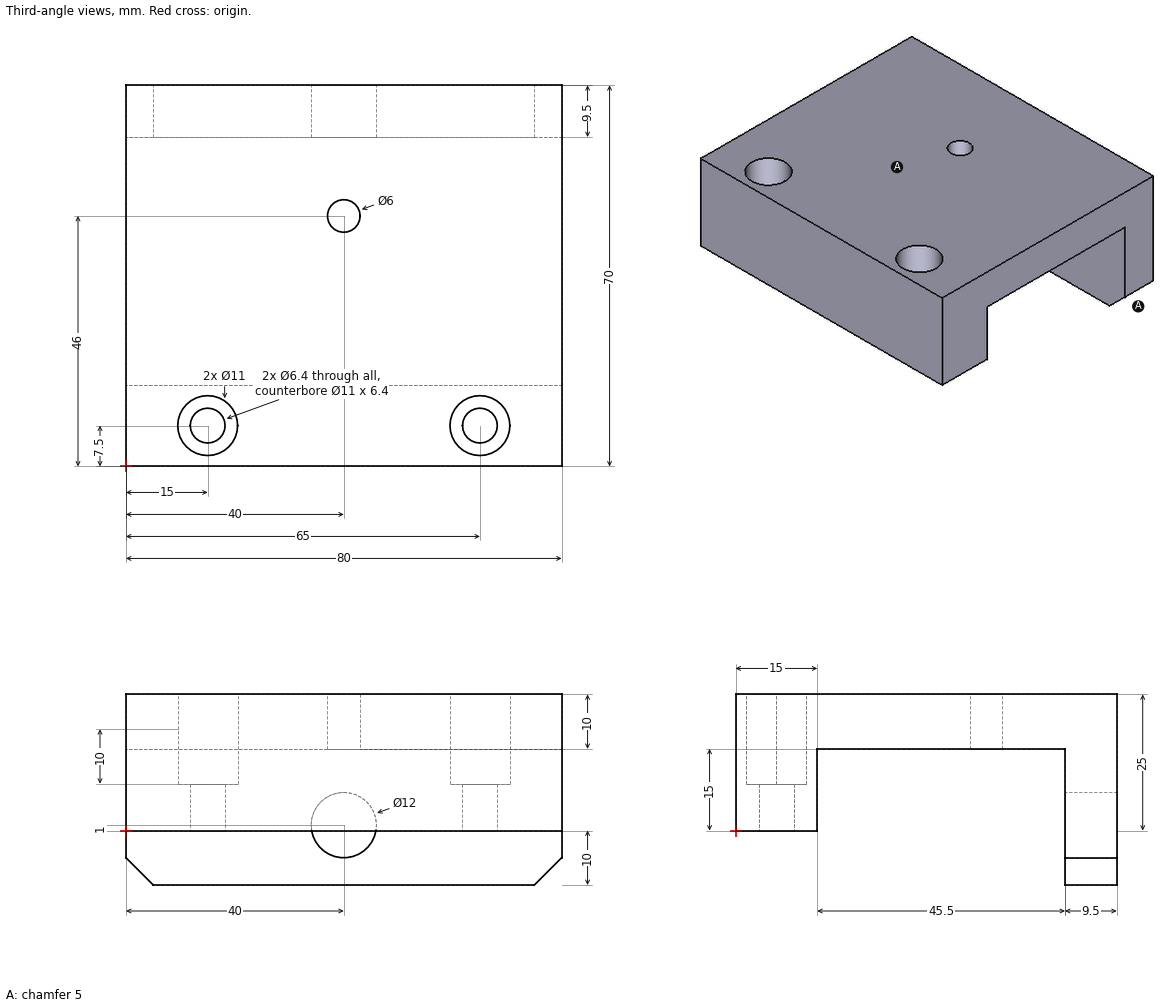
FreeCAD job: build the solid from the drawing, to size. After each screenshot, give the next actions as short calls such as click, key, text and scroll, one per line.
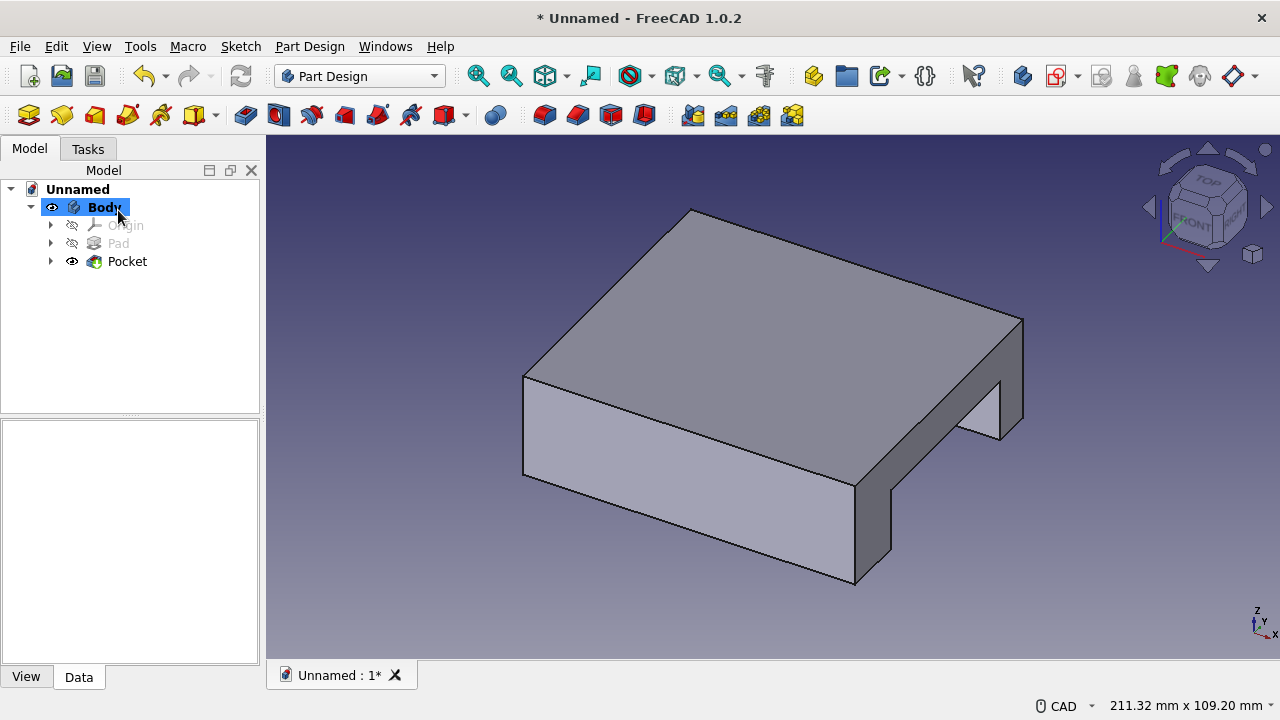
click(773, 347)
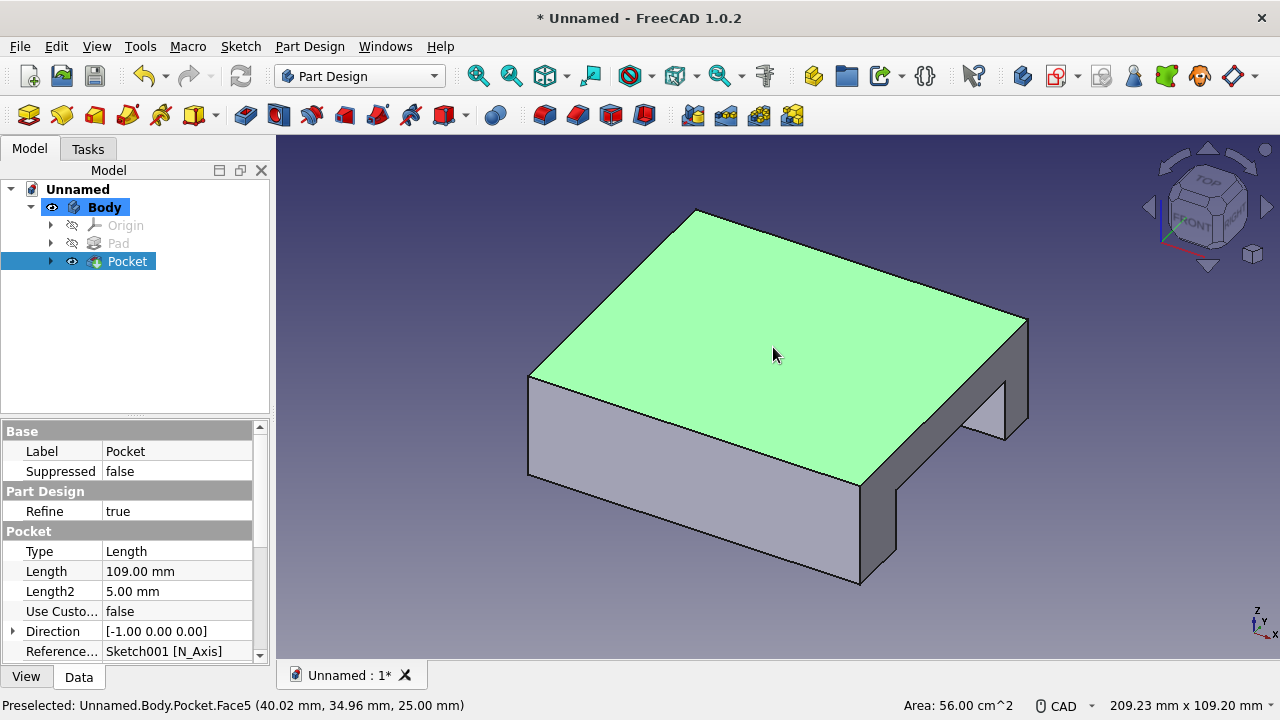
click(1056, 76)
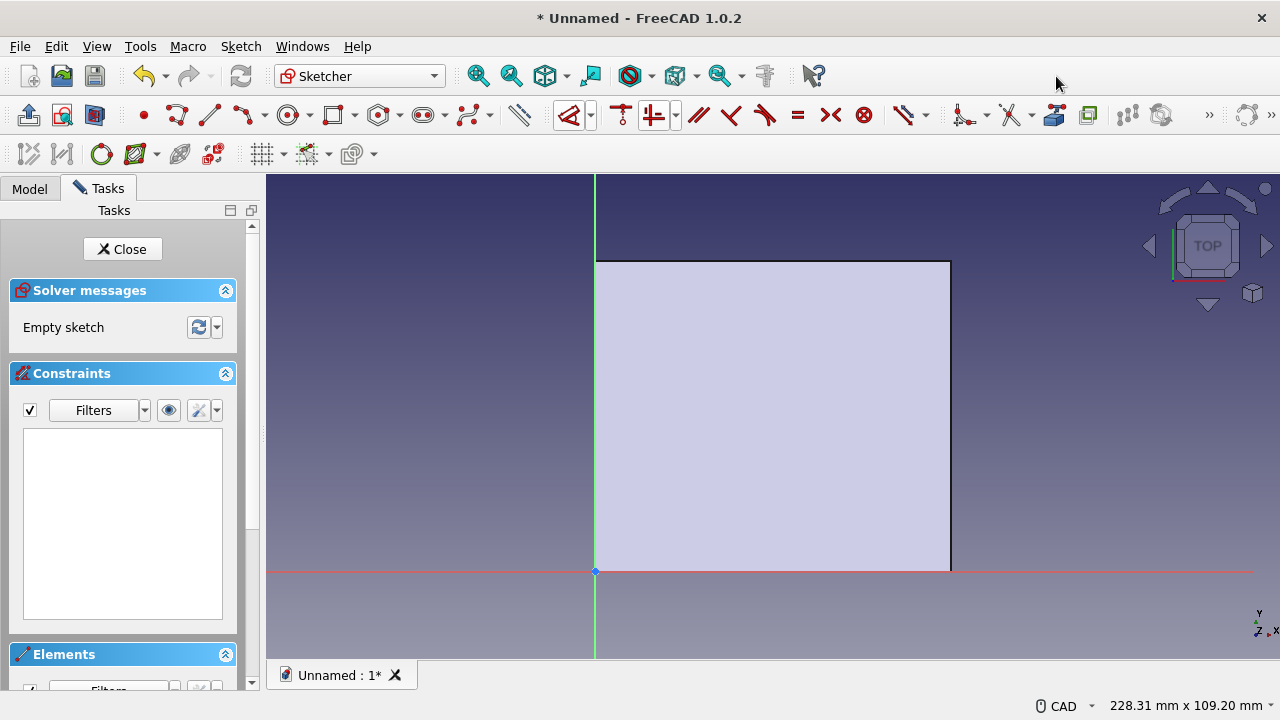
scroll(798, 631, up, 3)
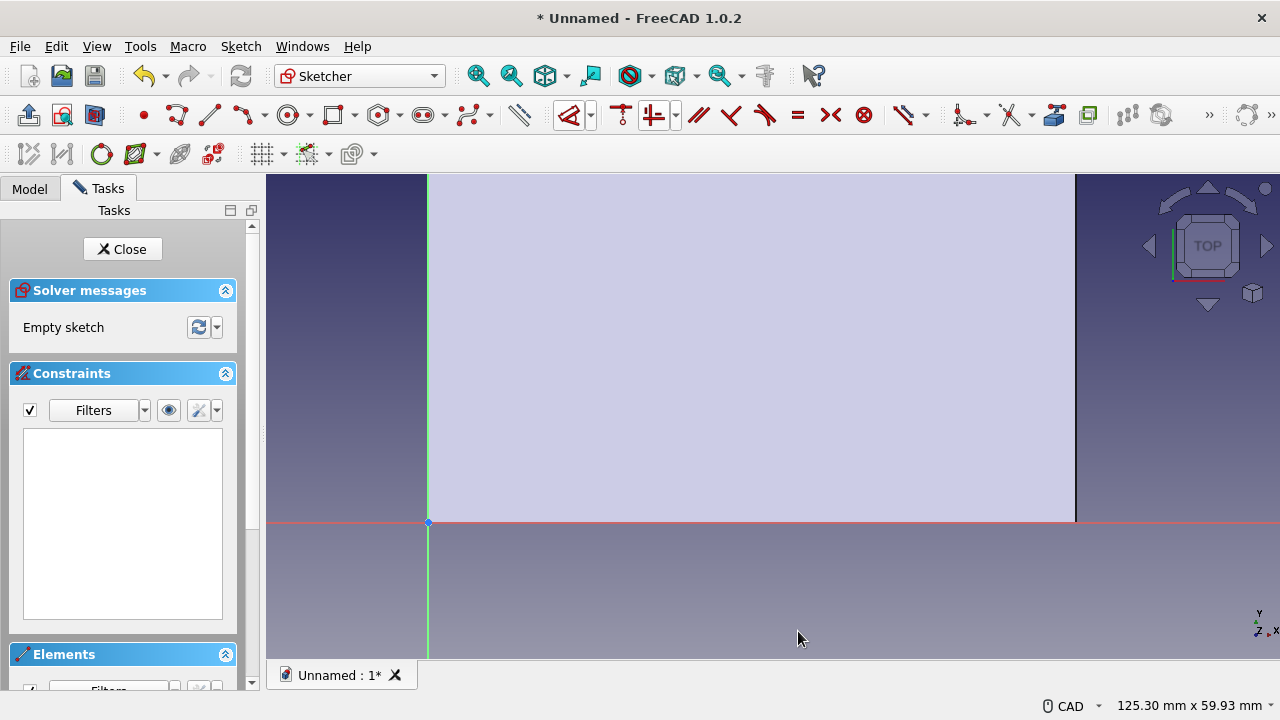
click(288, 116)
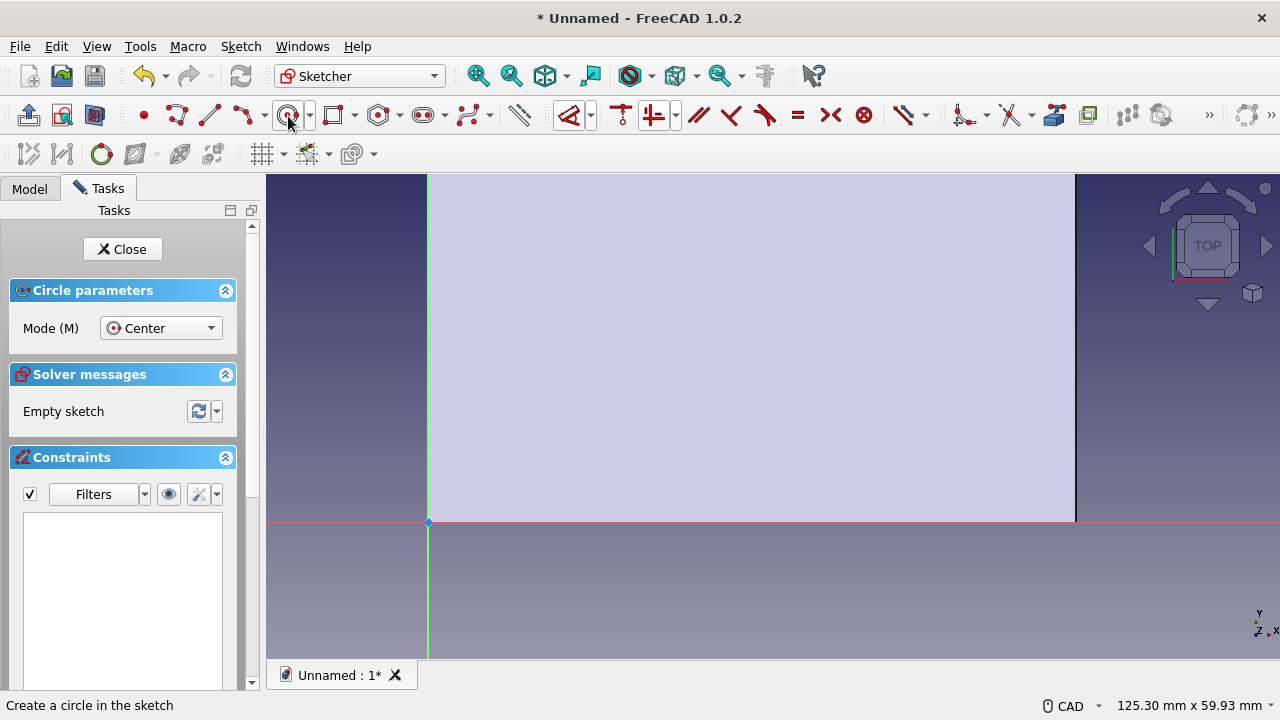
click(550, 462)
move(568, 444)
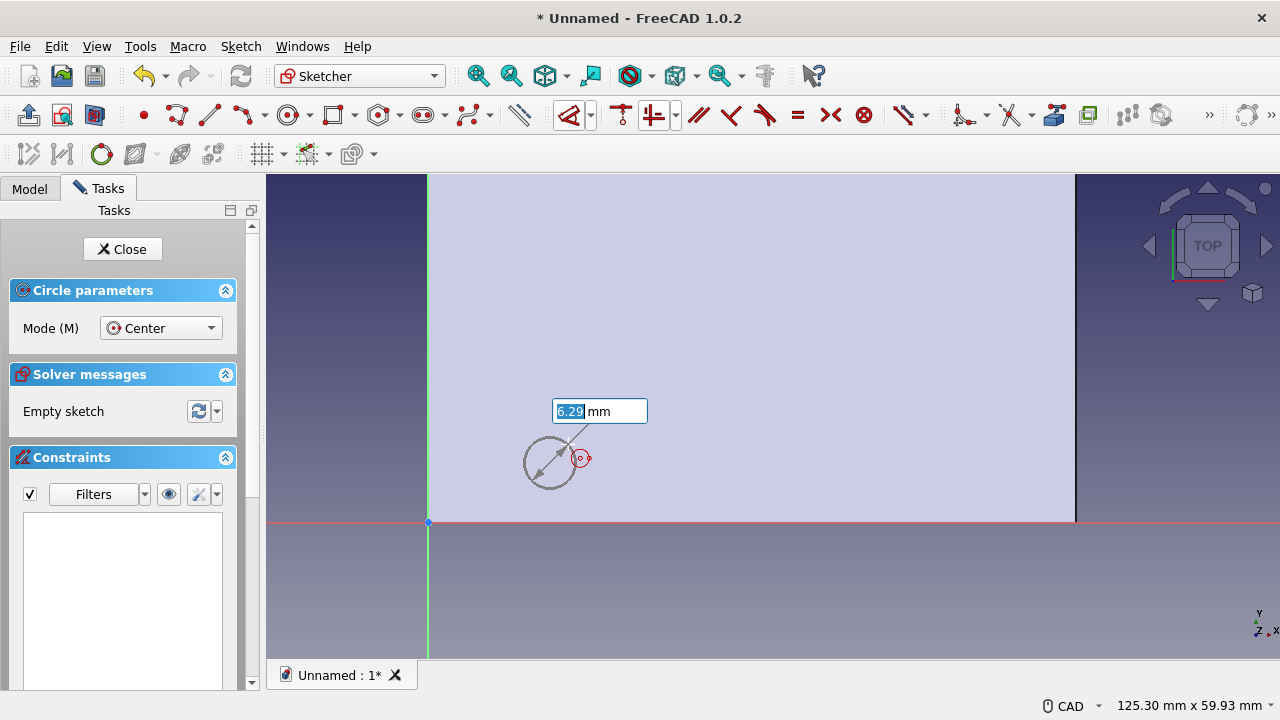
text(6.4)
key(Return)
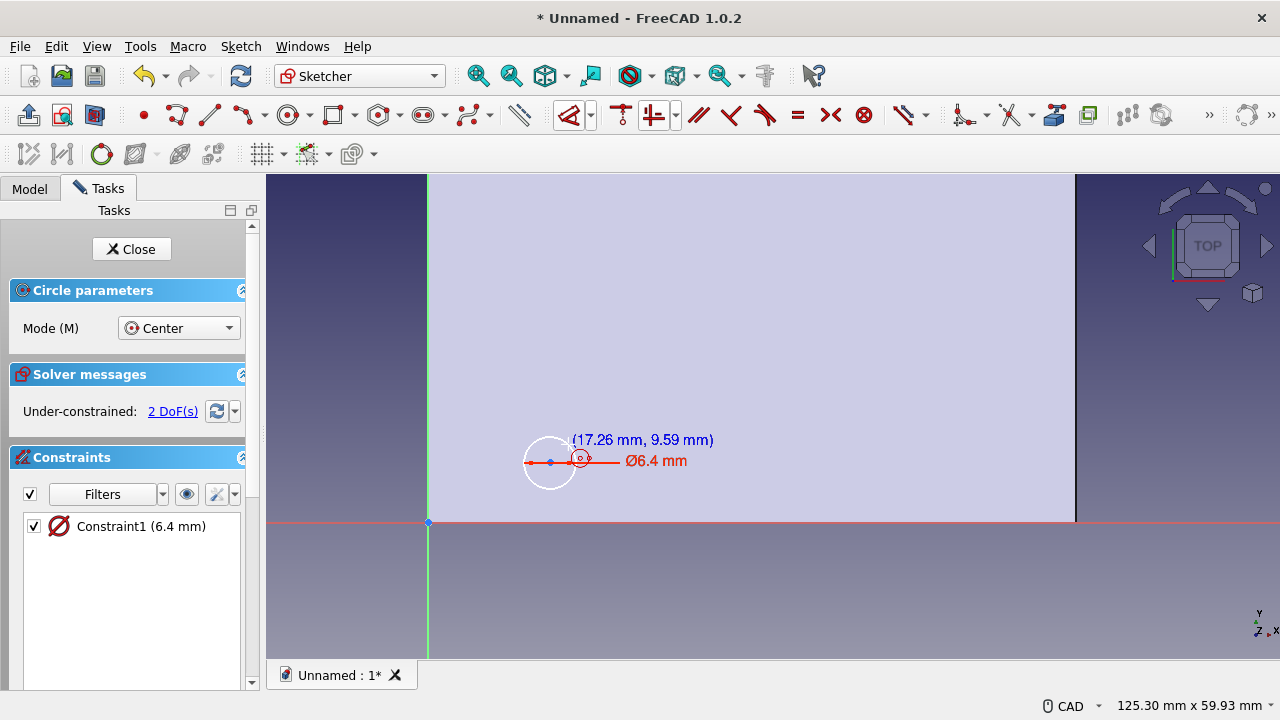
click(954, 462)
move(973, 444)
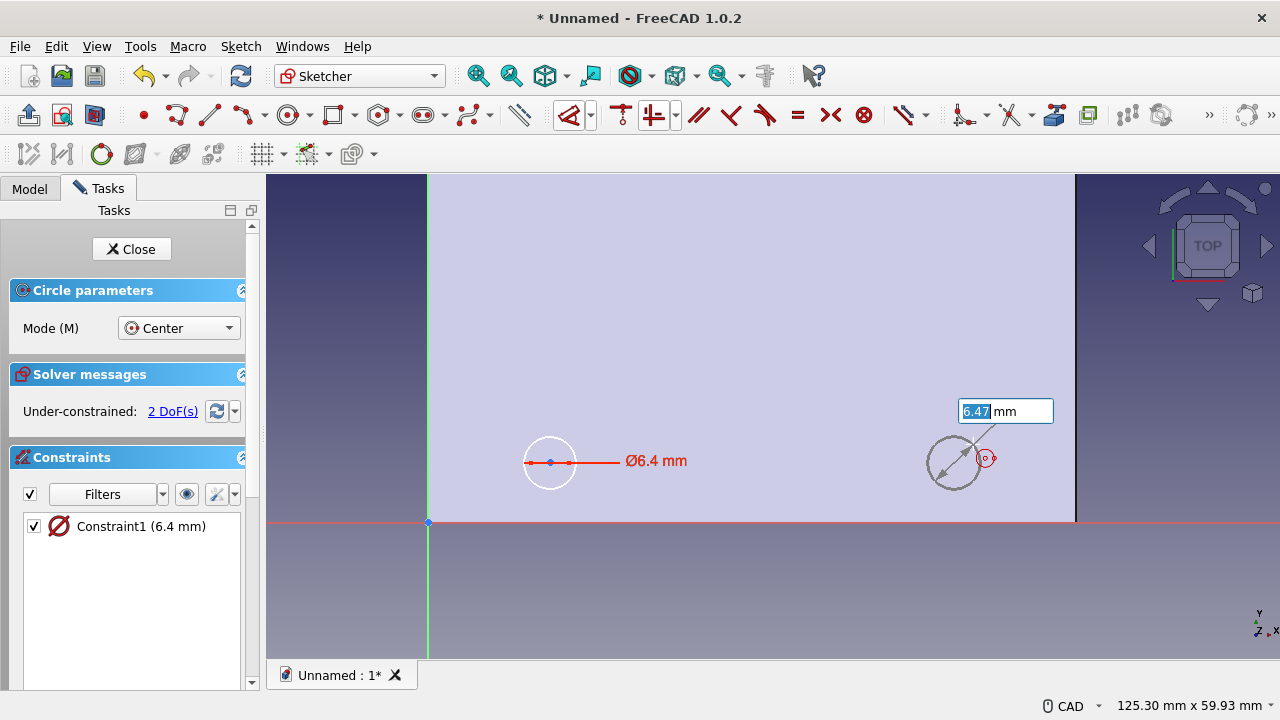
text(6.4)
key(Return)
key(Escape)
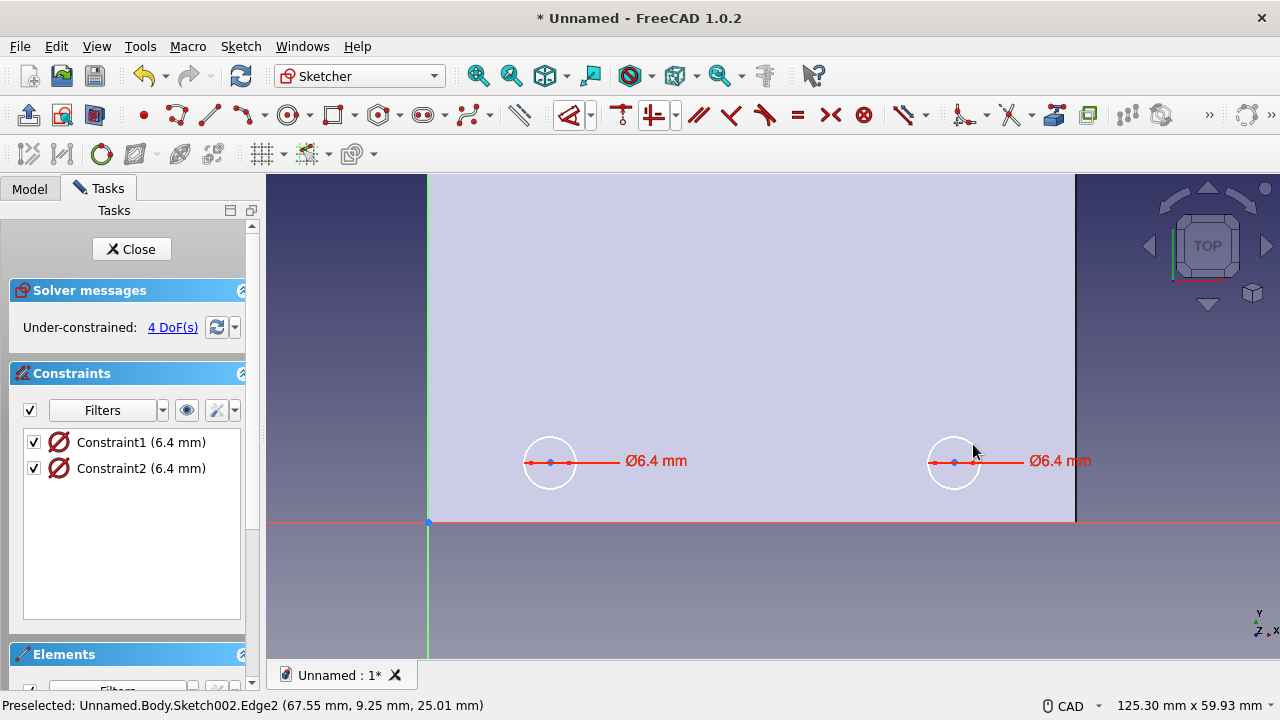
click(550, 463)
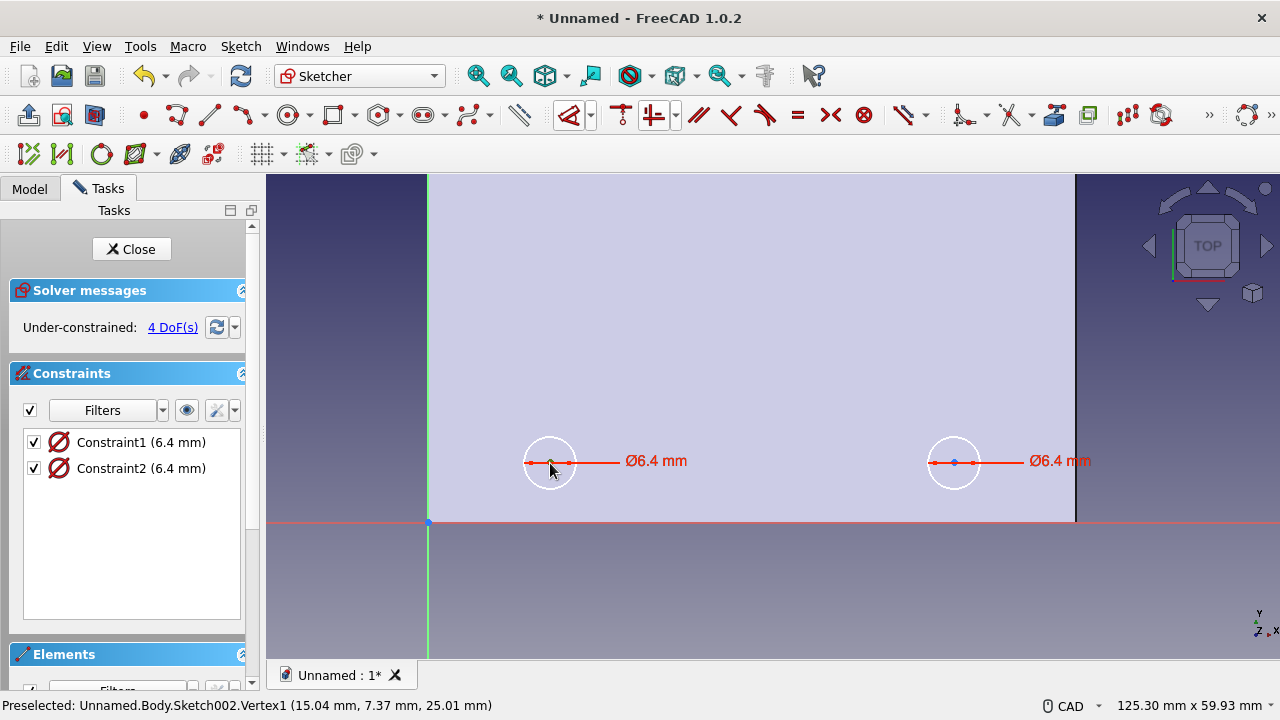
click(954, 463)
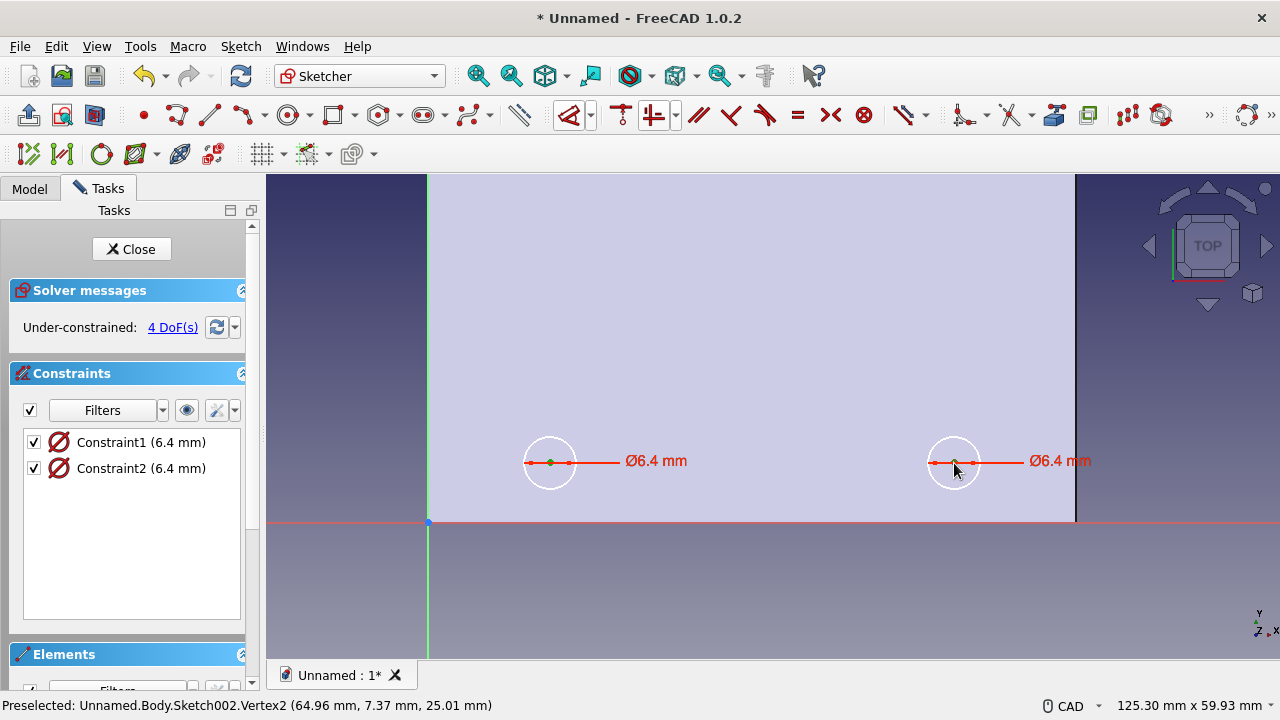
click(676, 116)